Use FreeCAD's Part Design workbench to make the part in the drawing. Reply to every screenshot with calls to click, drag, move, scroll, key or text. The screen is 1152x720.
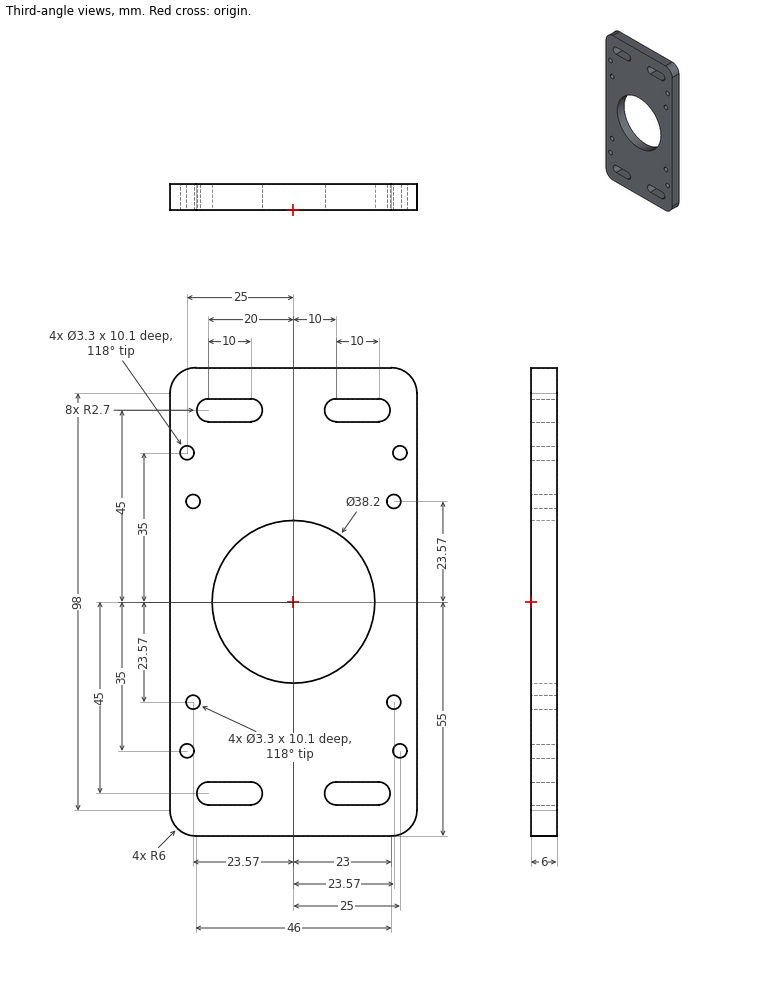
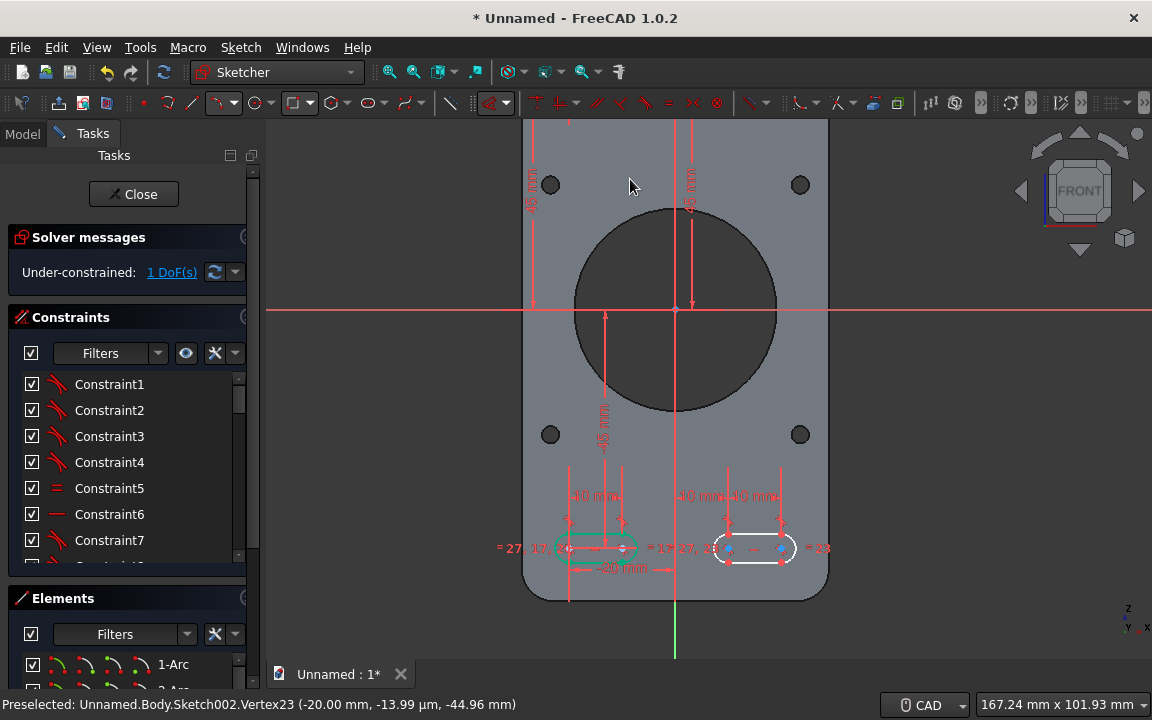
click(728, 549)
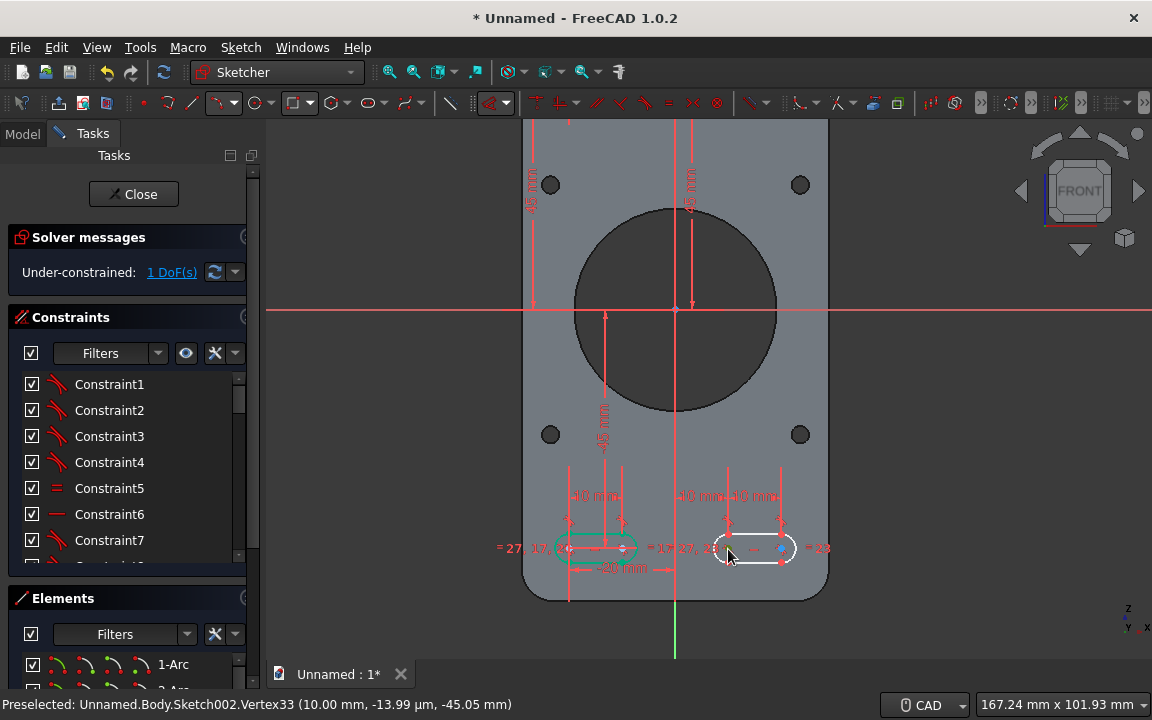
click(508, 104)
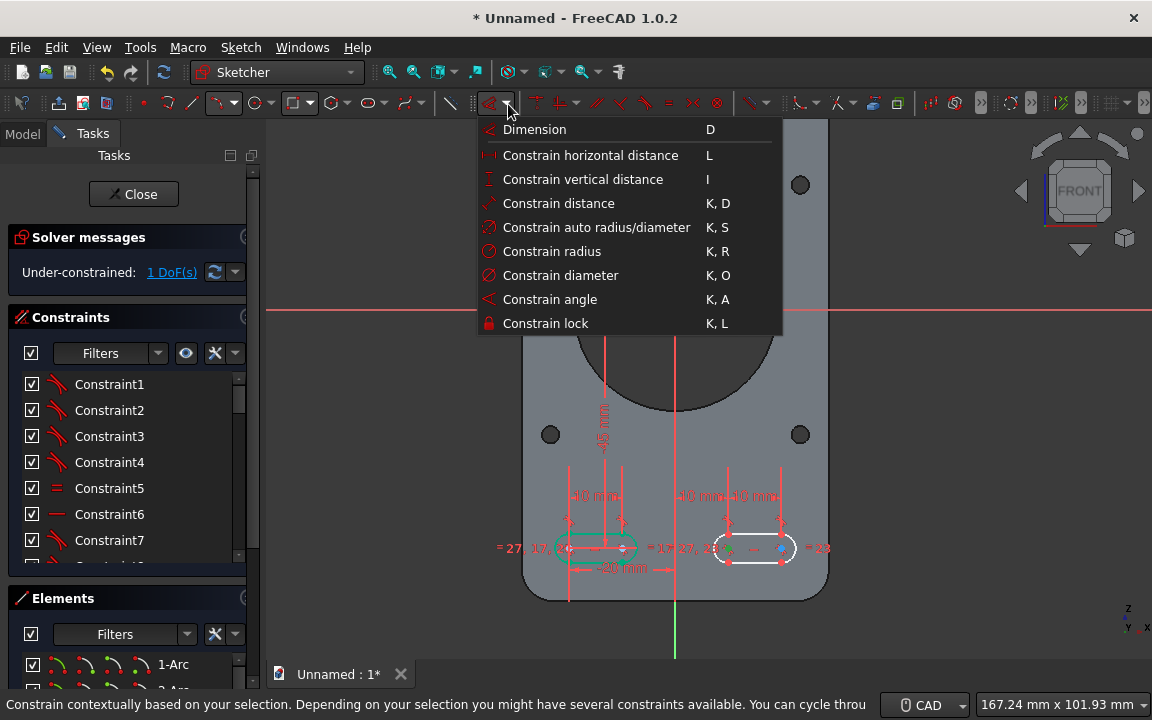
click(630, 179)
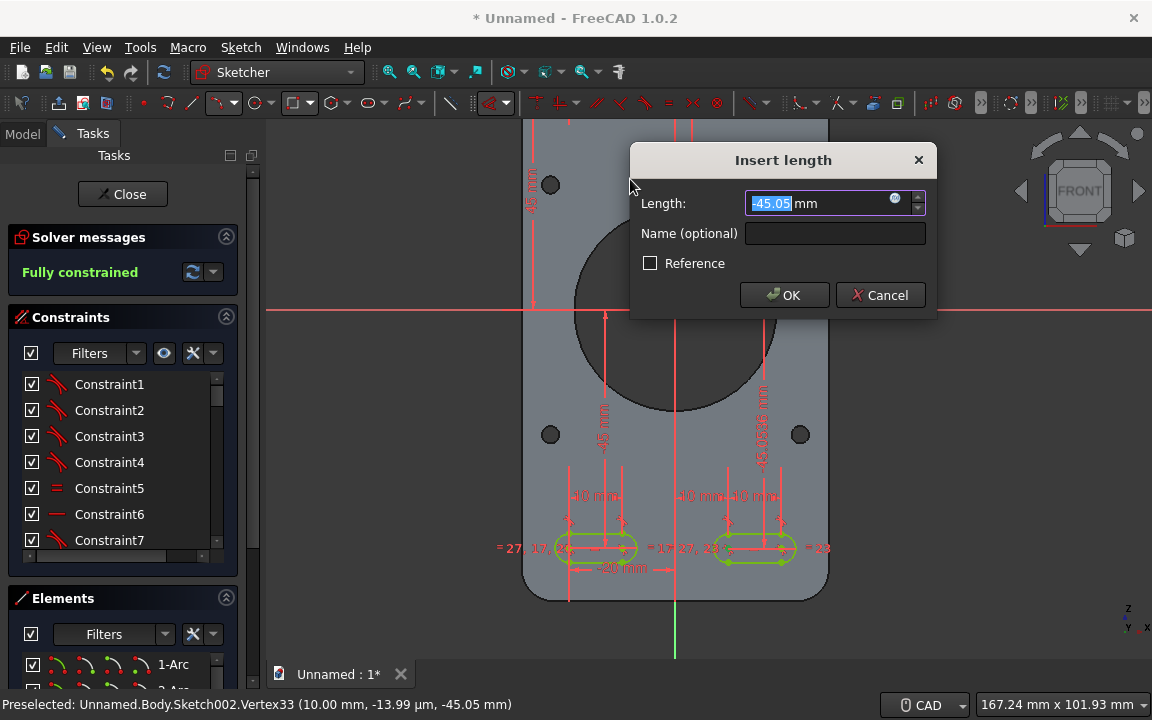
text(-45)
key(Return)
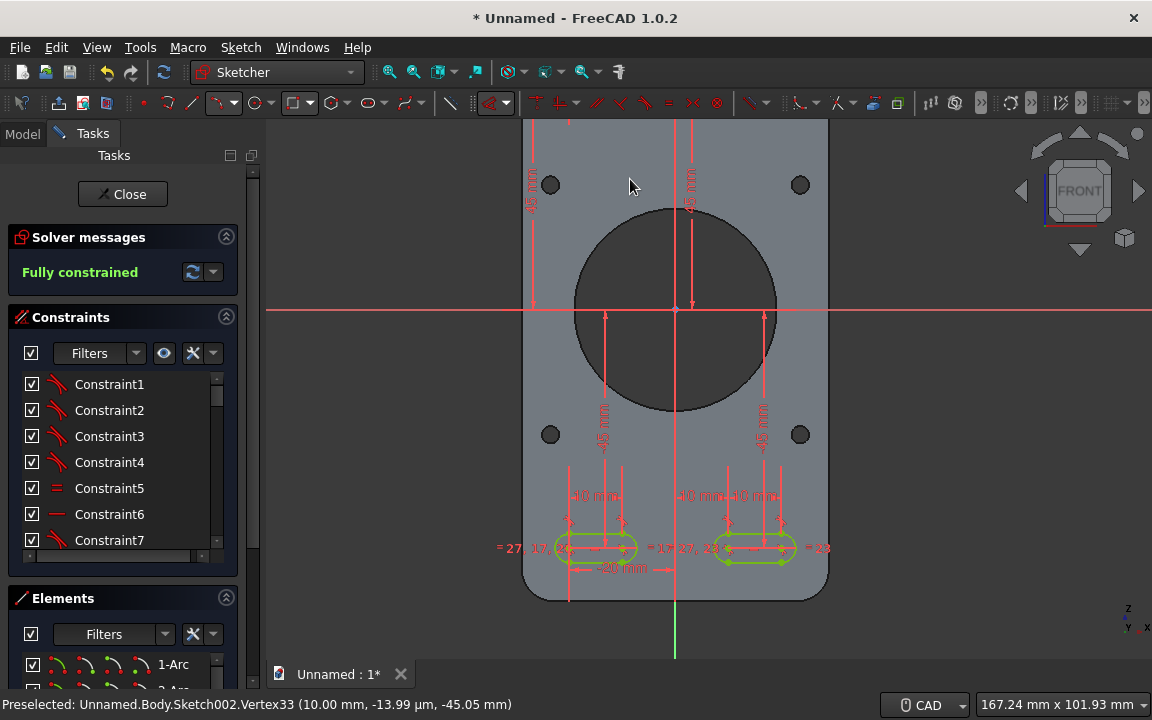
click(123, 194)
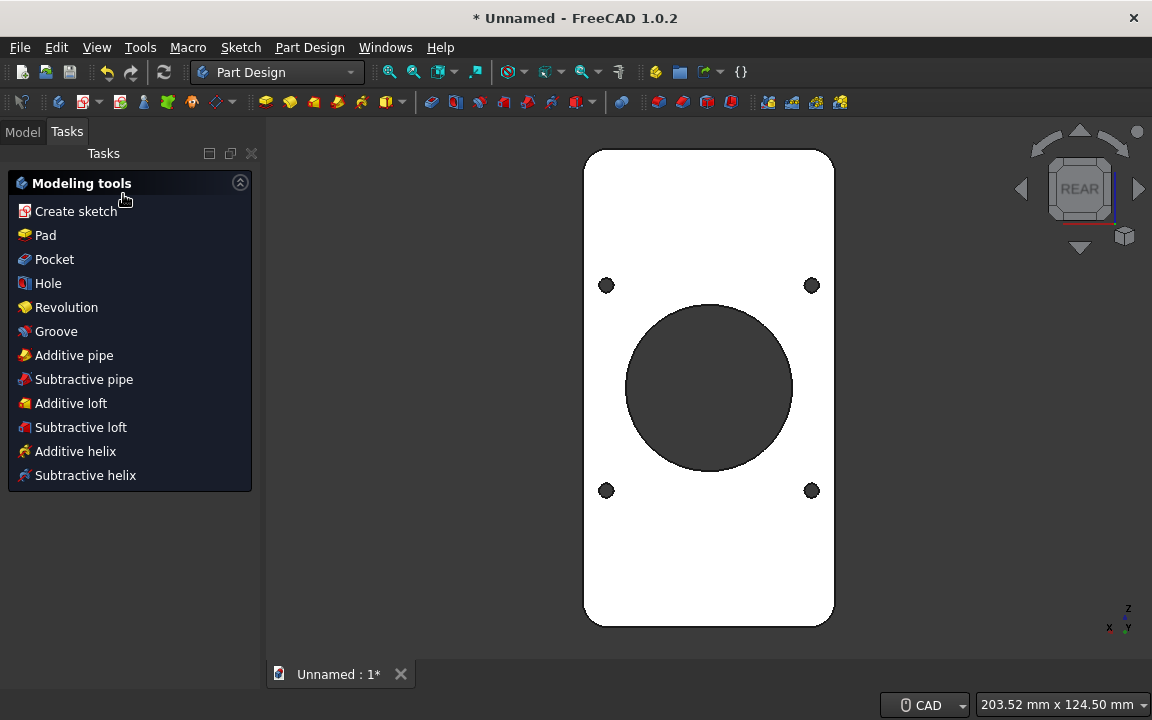
click(432, 102)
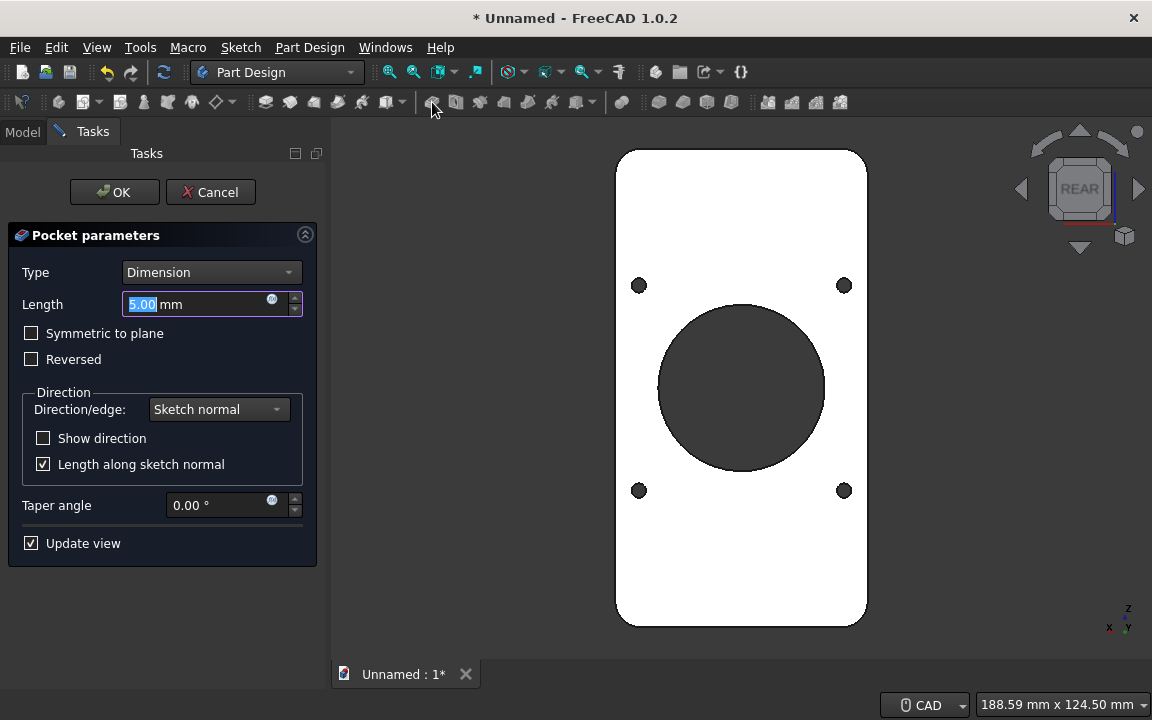
click(212, 272)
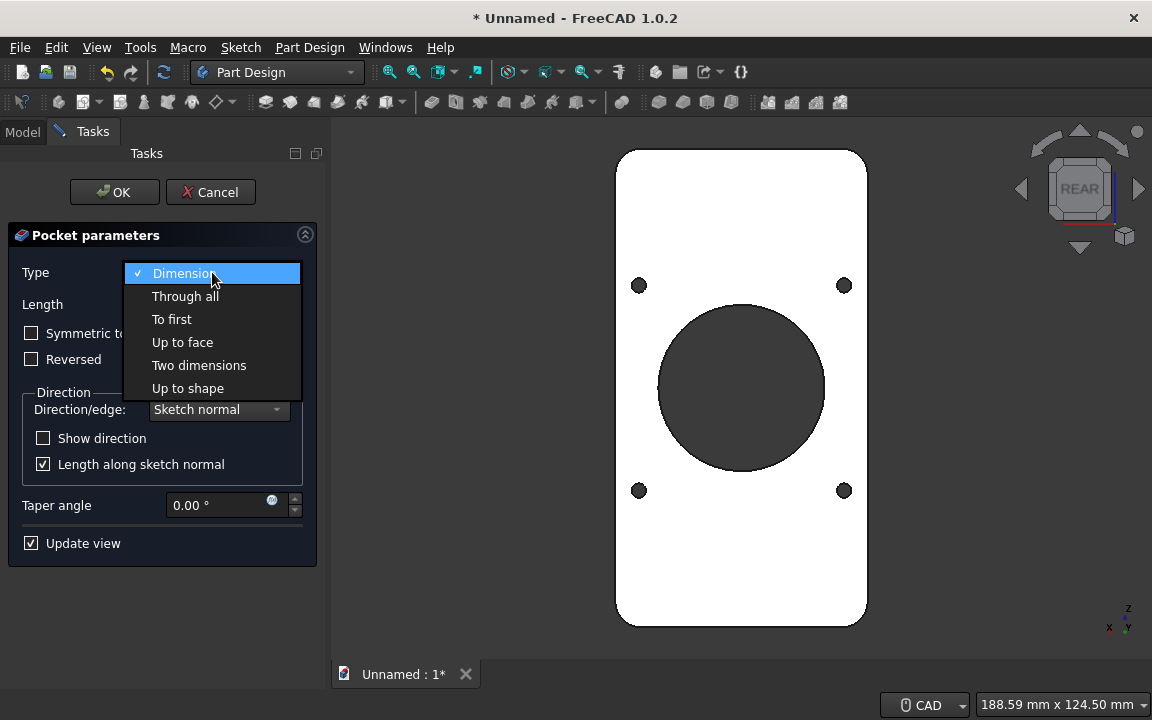
click(212, 296)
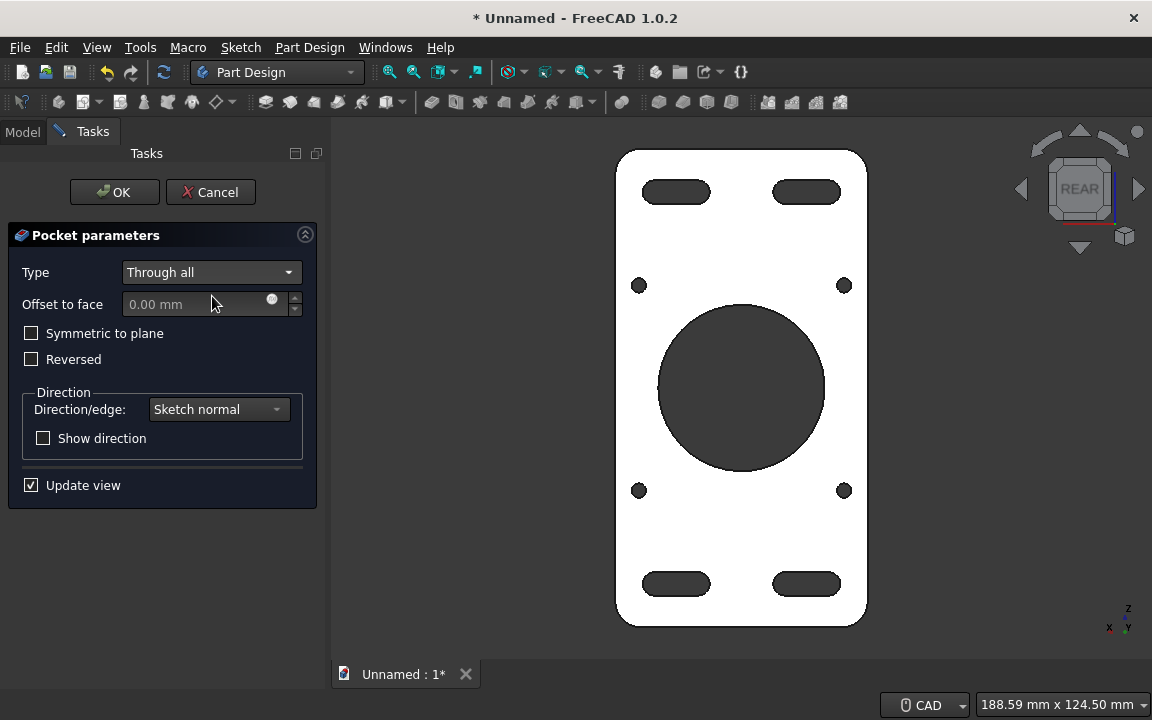
click(115, 192)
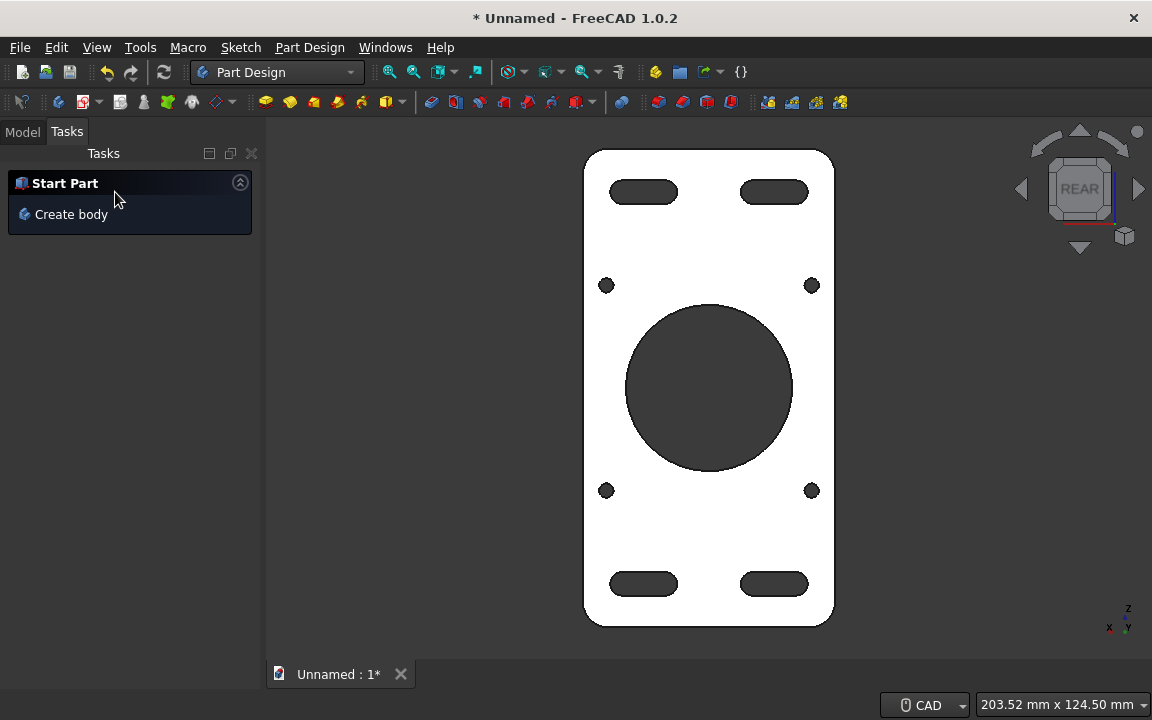
click(84, 102)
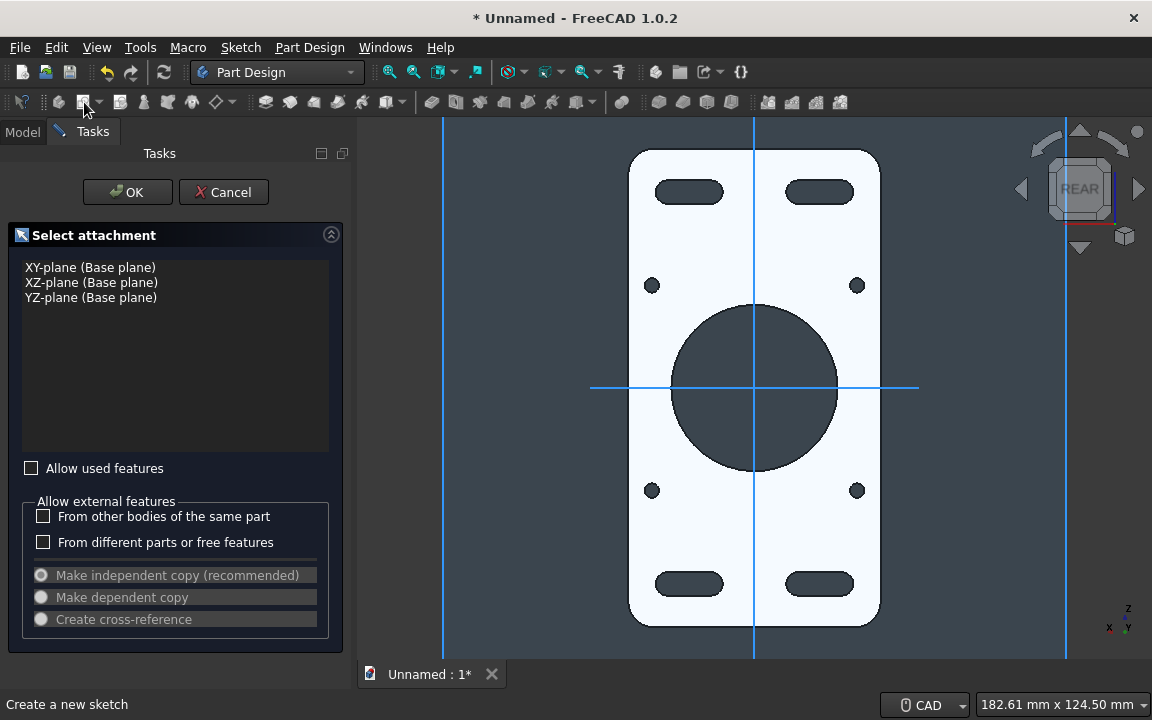
click(82, 282)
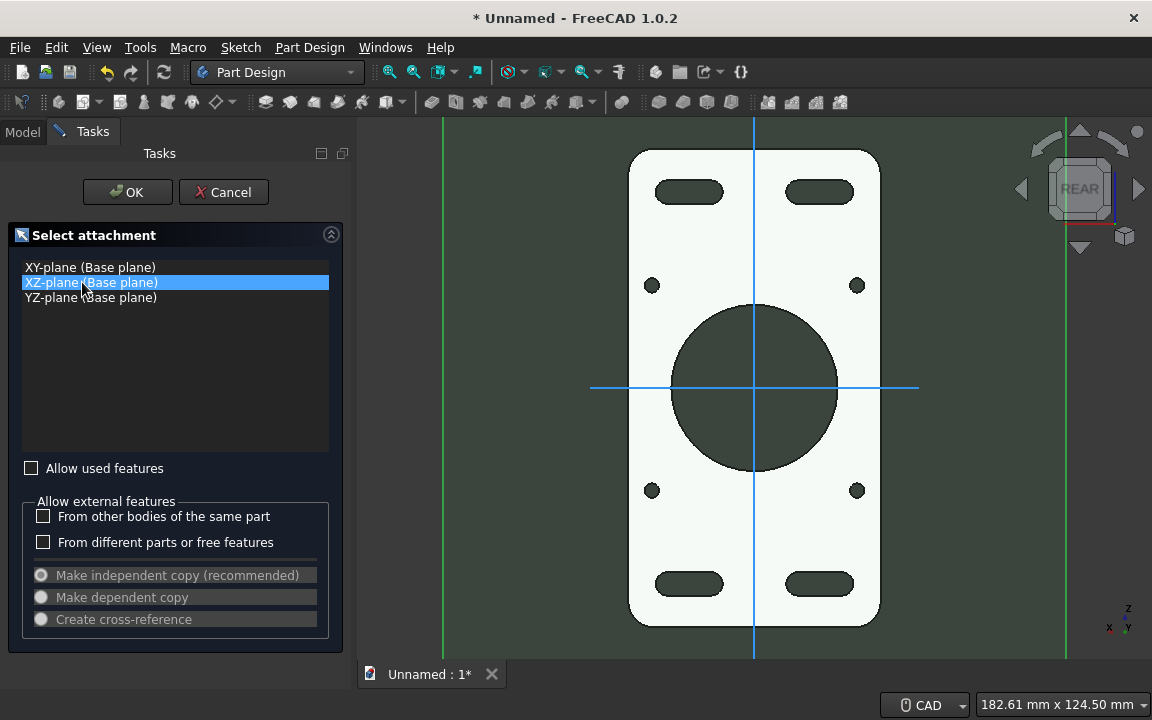
click(128, 192)